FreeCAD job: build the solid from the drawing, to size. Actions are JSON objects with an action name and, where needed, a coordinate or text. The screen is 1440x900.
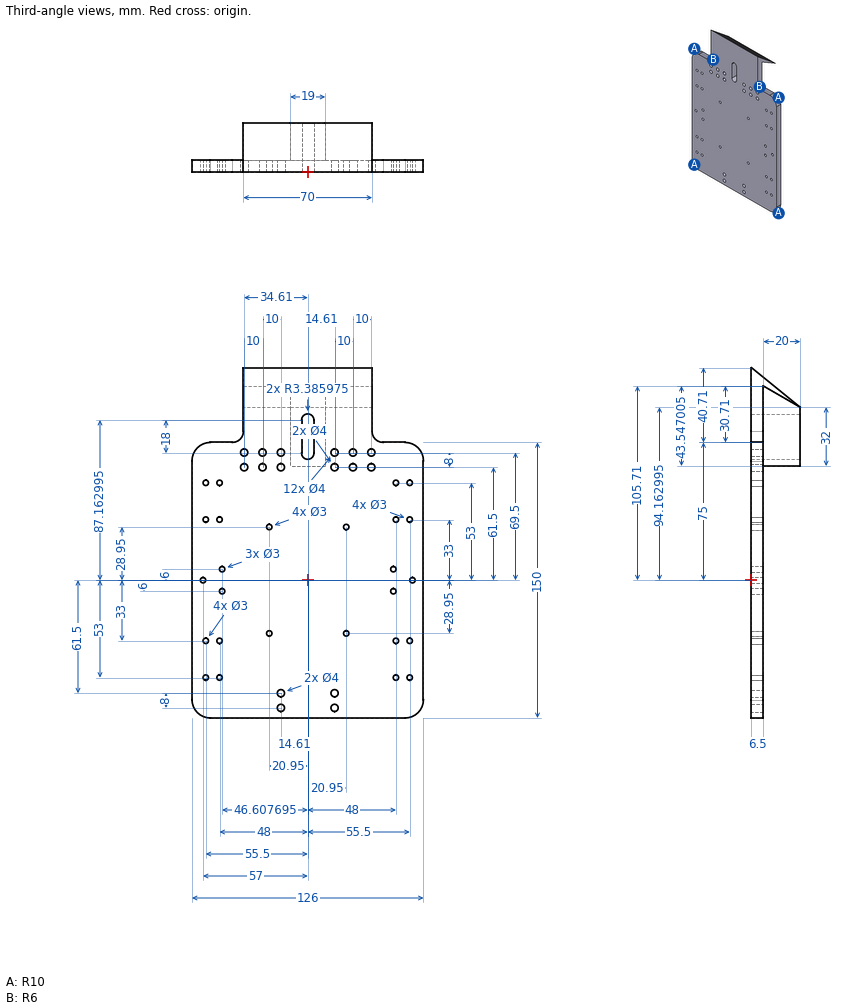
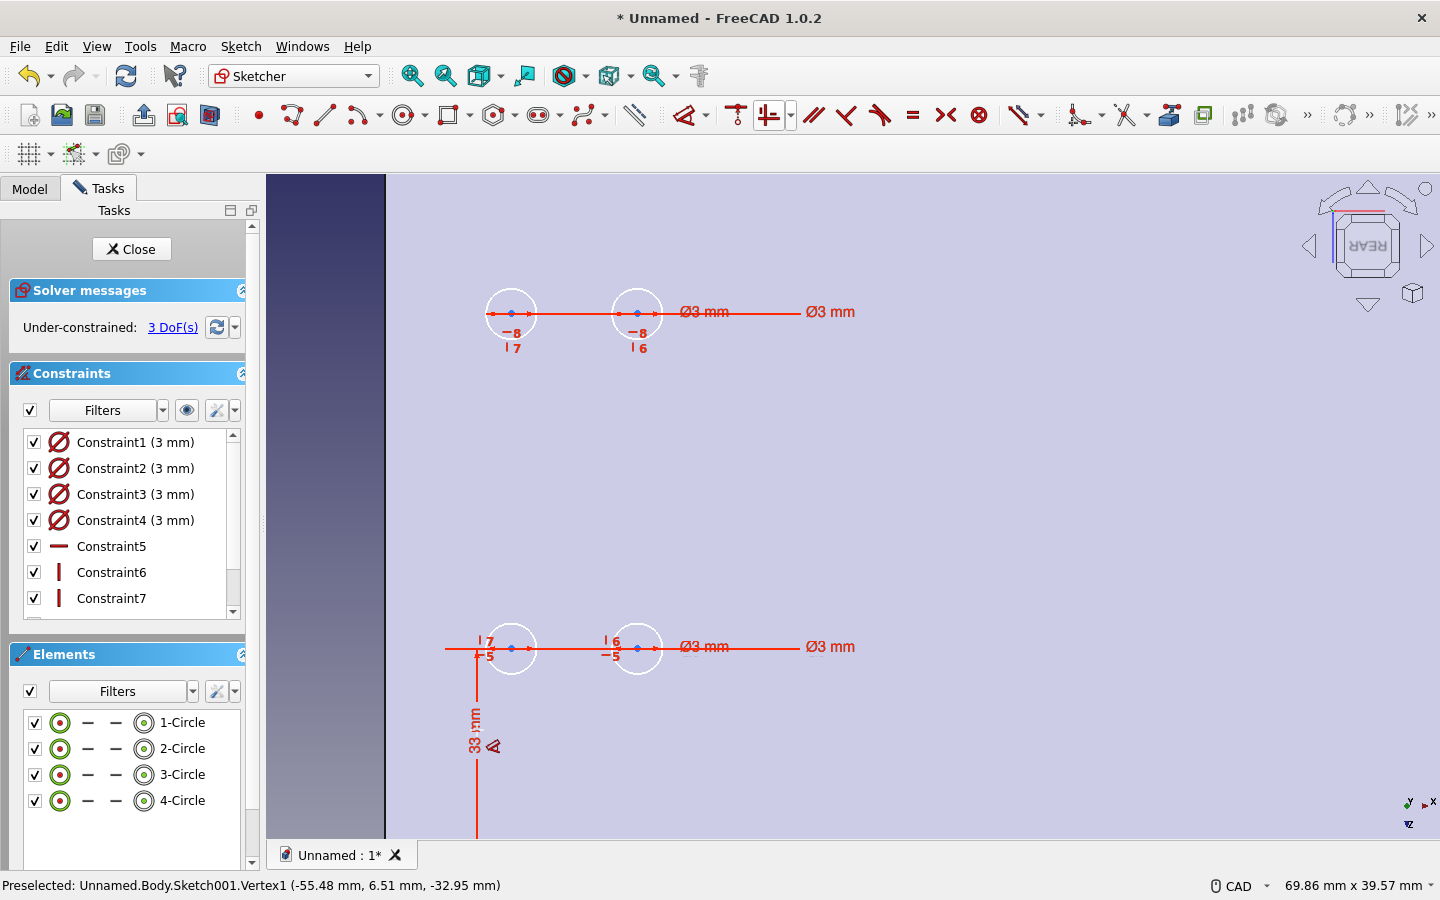
{"action": "left_click", "coordinate": [637, 649]}
{"action": "left_click", "coordinate": [956, 615]}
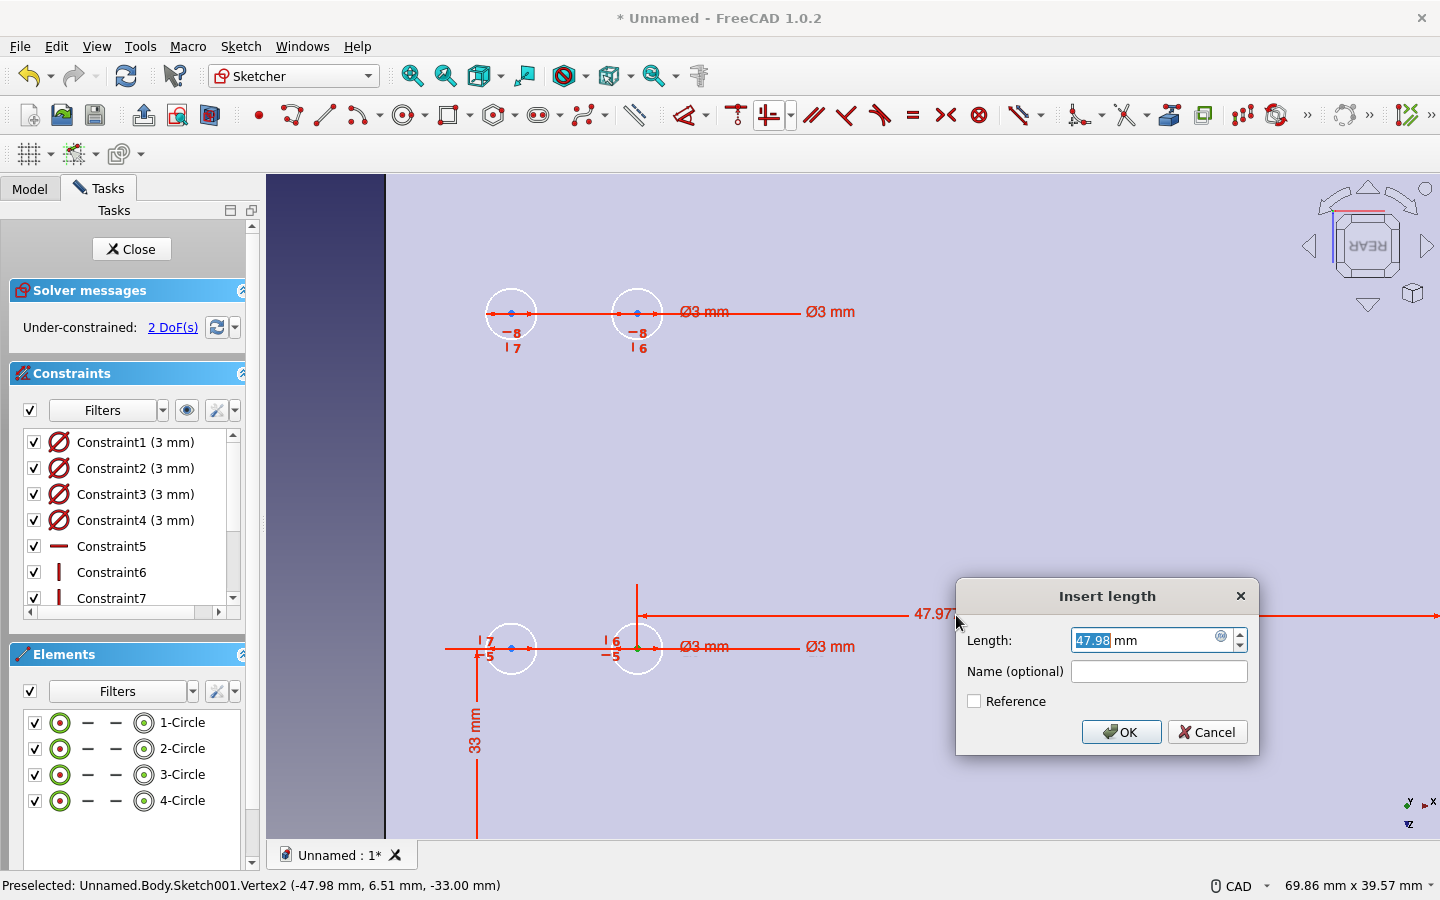
{"action": "type", "text": "48"}
{"action": "key", "text": "Return"}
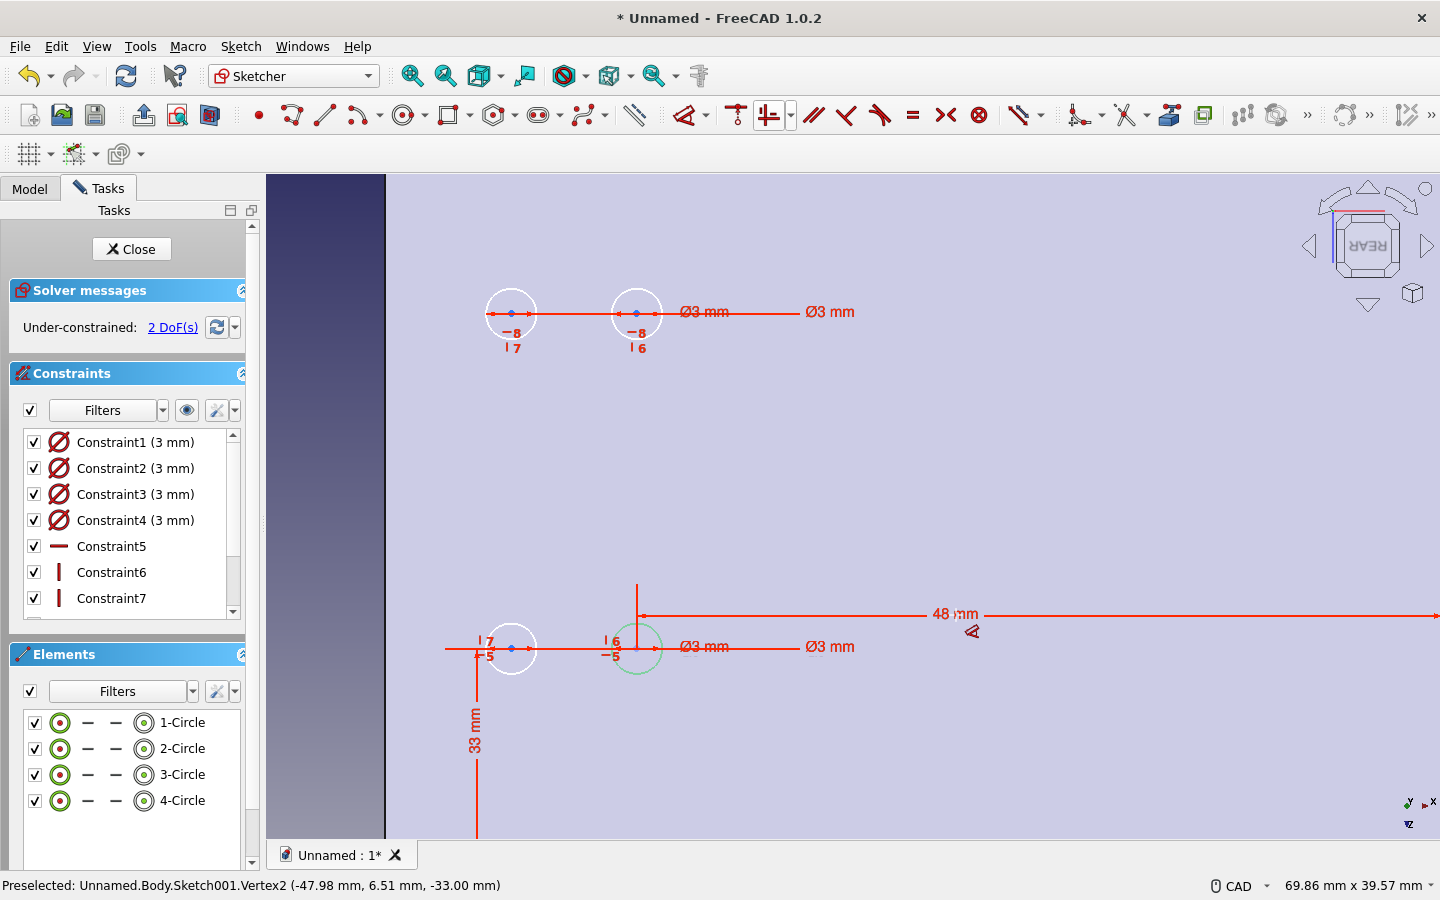
{"action": "left_click", "coordinate": [637, 314]}
{"action": "left_click", "coordinate": [603, 562]}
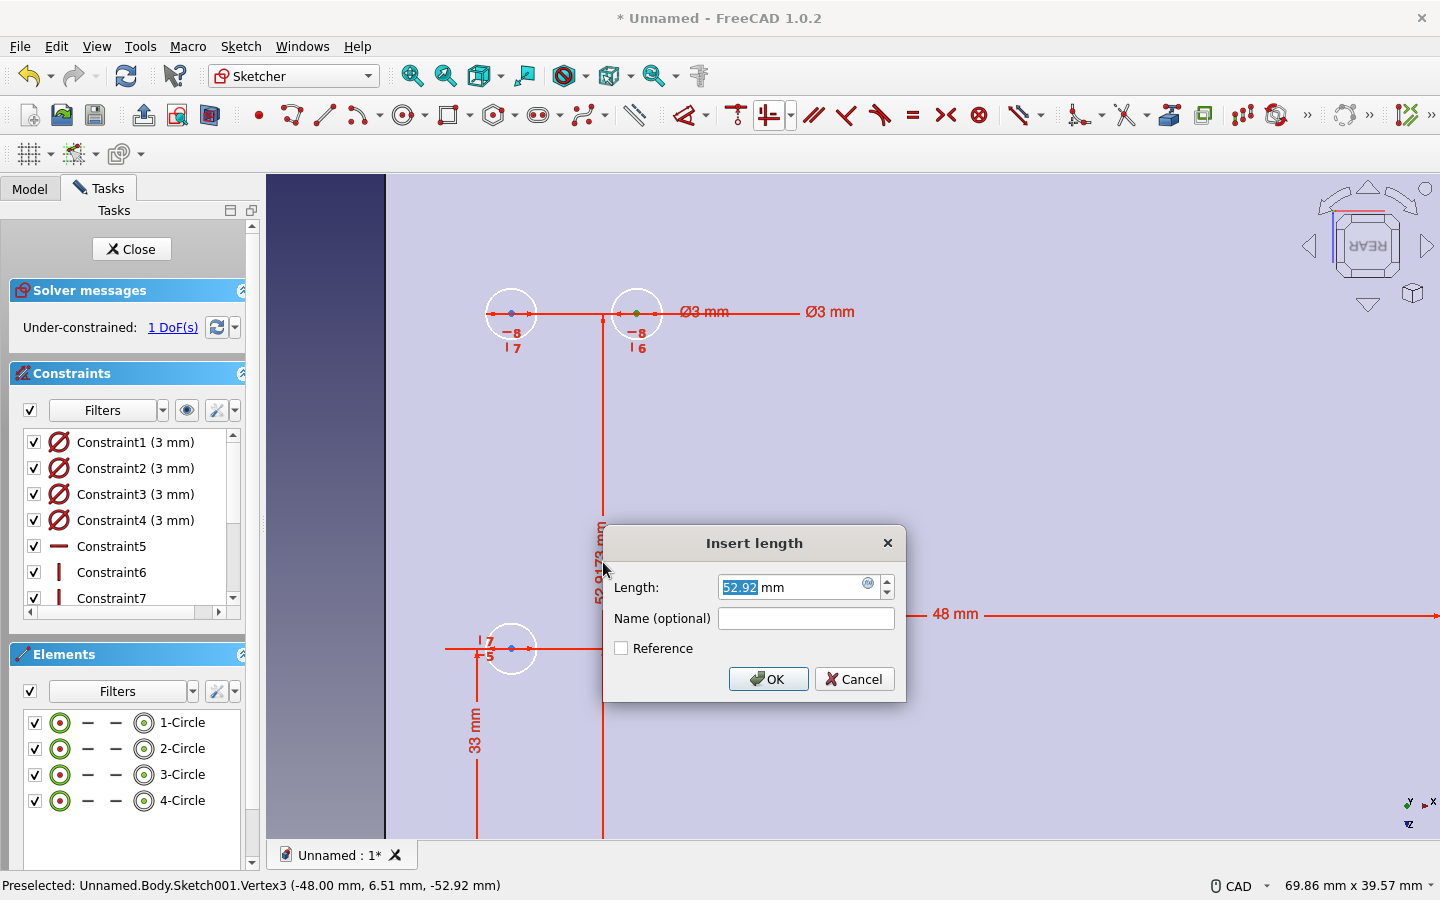
{"action": "type", "text": "53"}
{"action": "key", "text": "Return"}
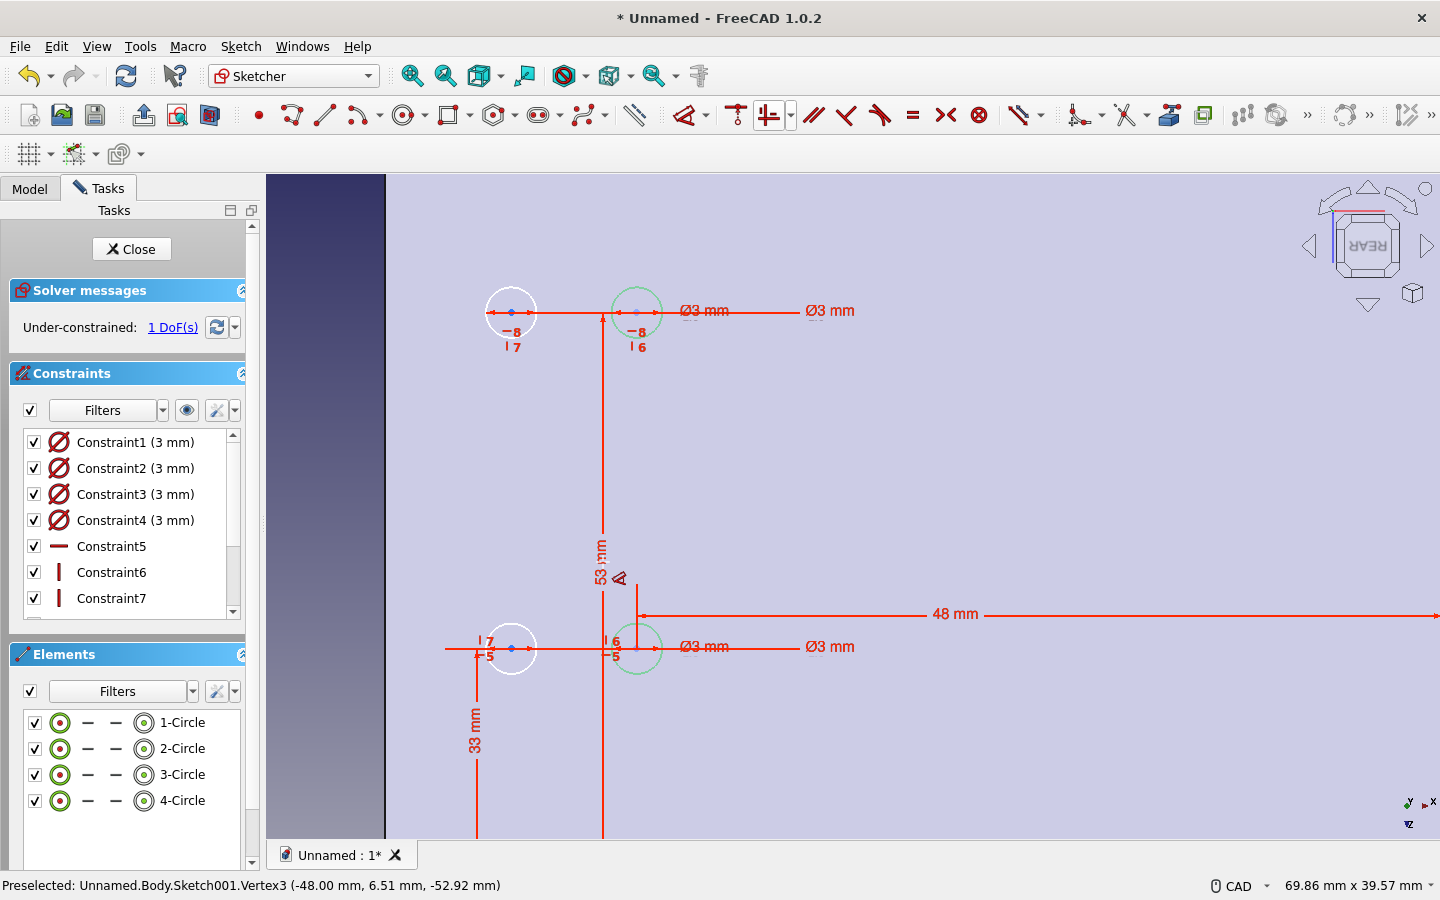
{"action": "left_click", "coordinate": [511, 649]}
{"action": "left_click", "coordinate": [718, 615]}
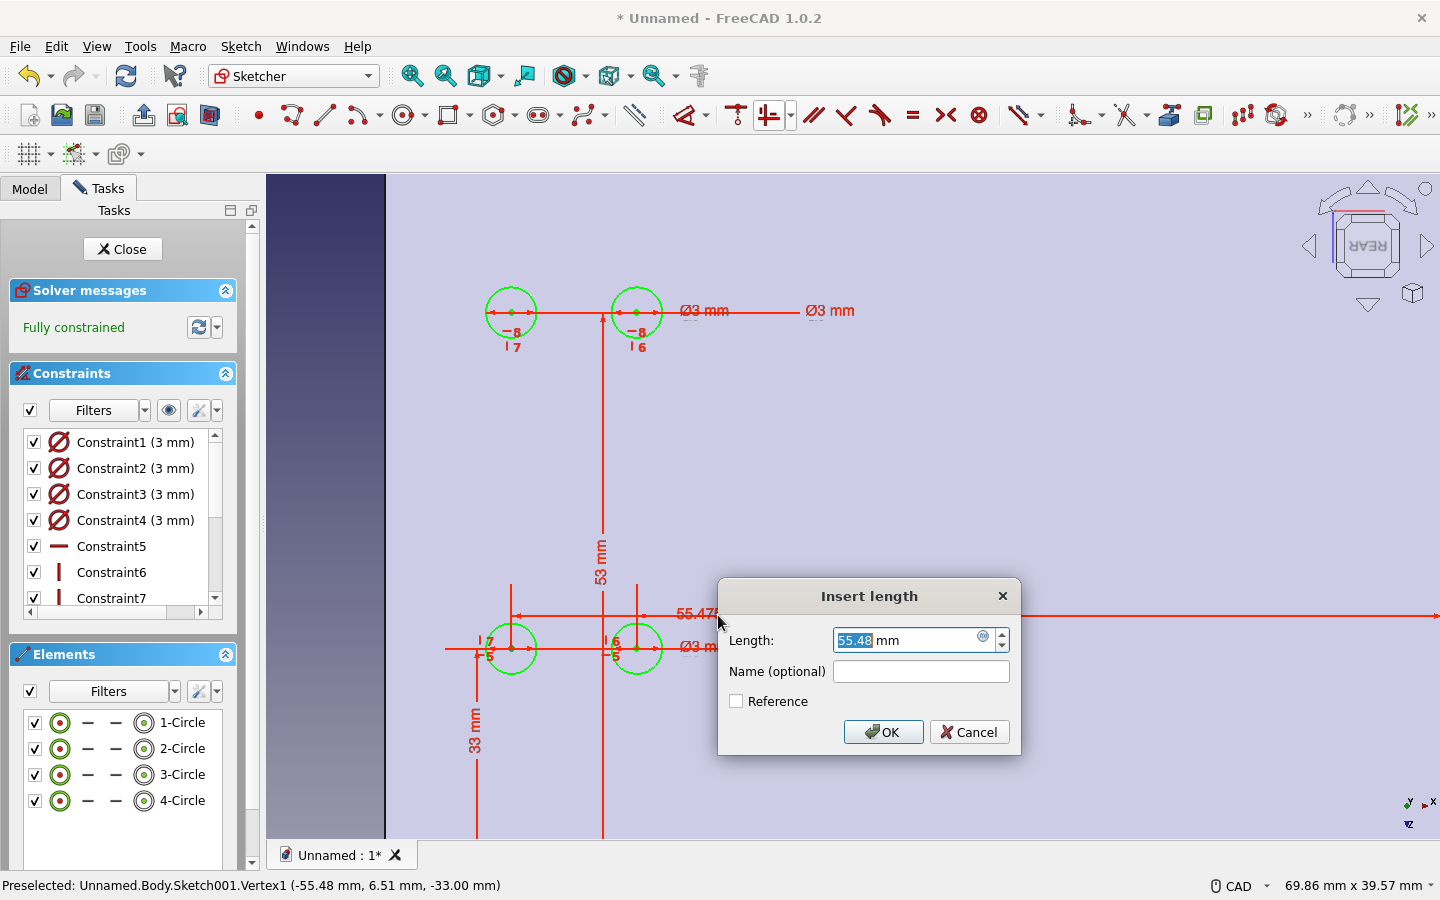
{"action": "type", "text": "55.5"}
{"action": "key", "text": "Return"}
{"action": "key", "text": "Escape"}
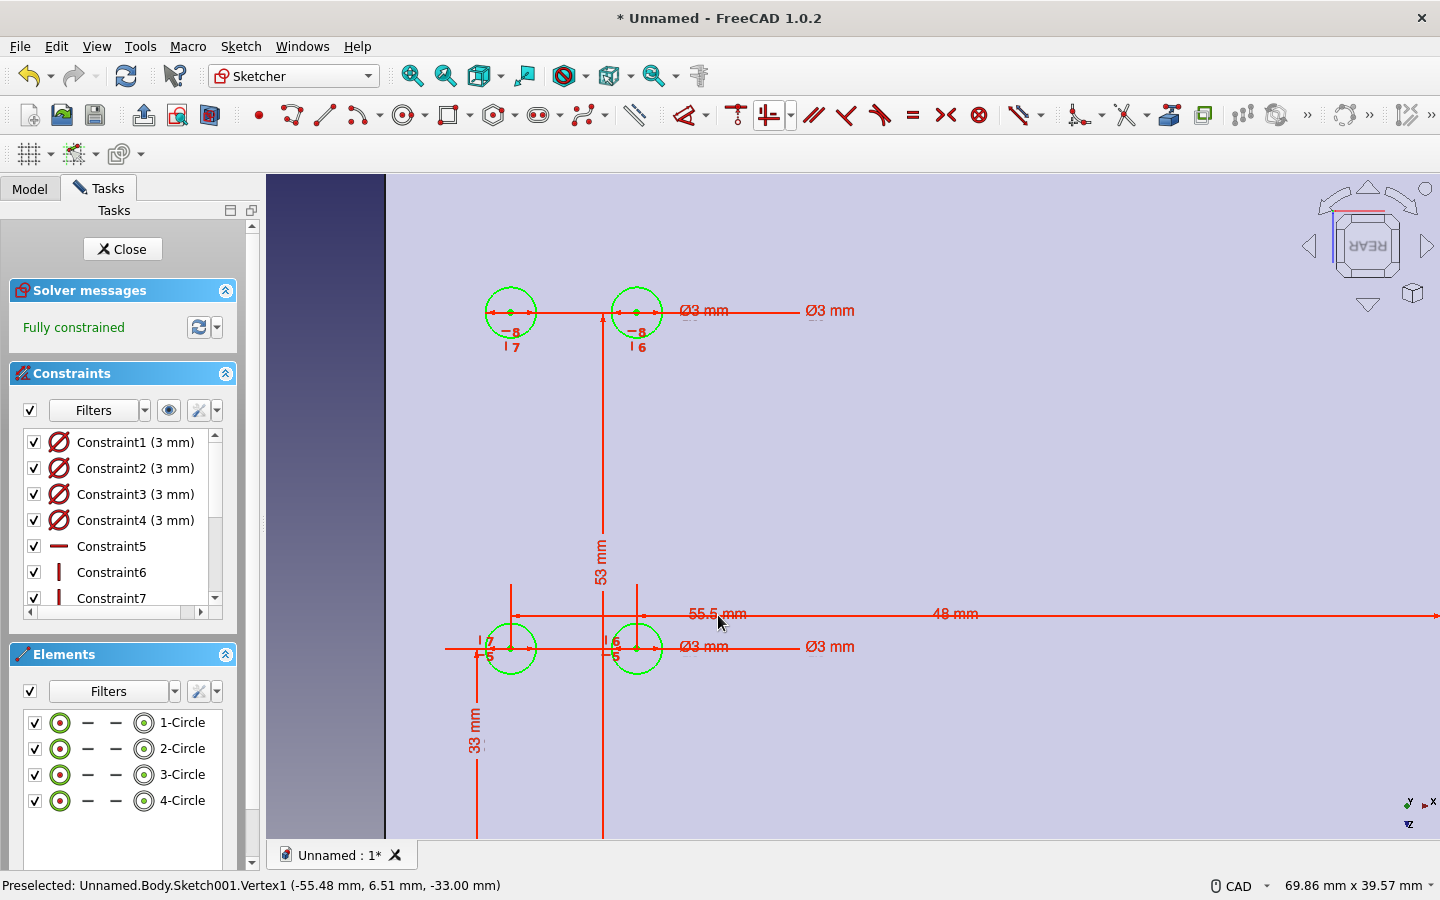
{"action": "left_click", "coordinate": [123, 249]}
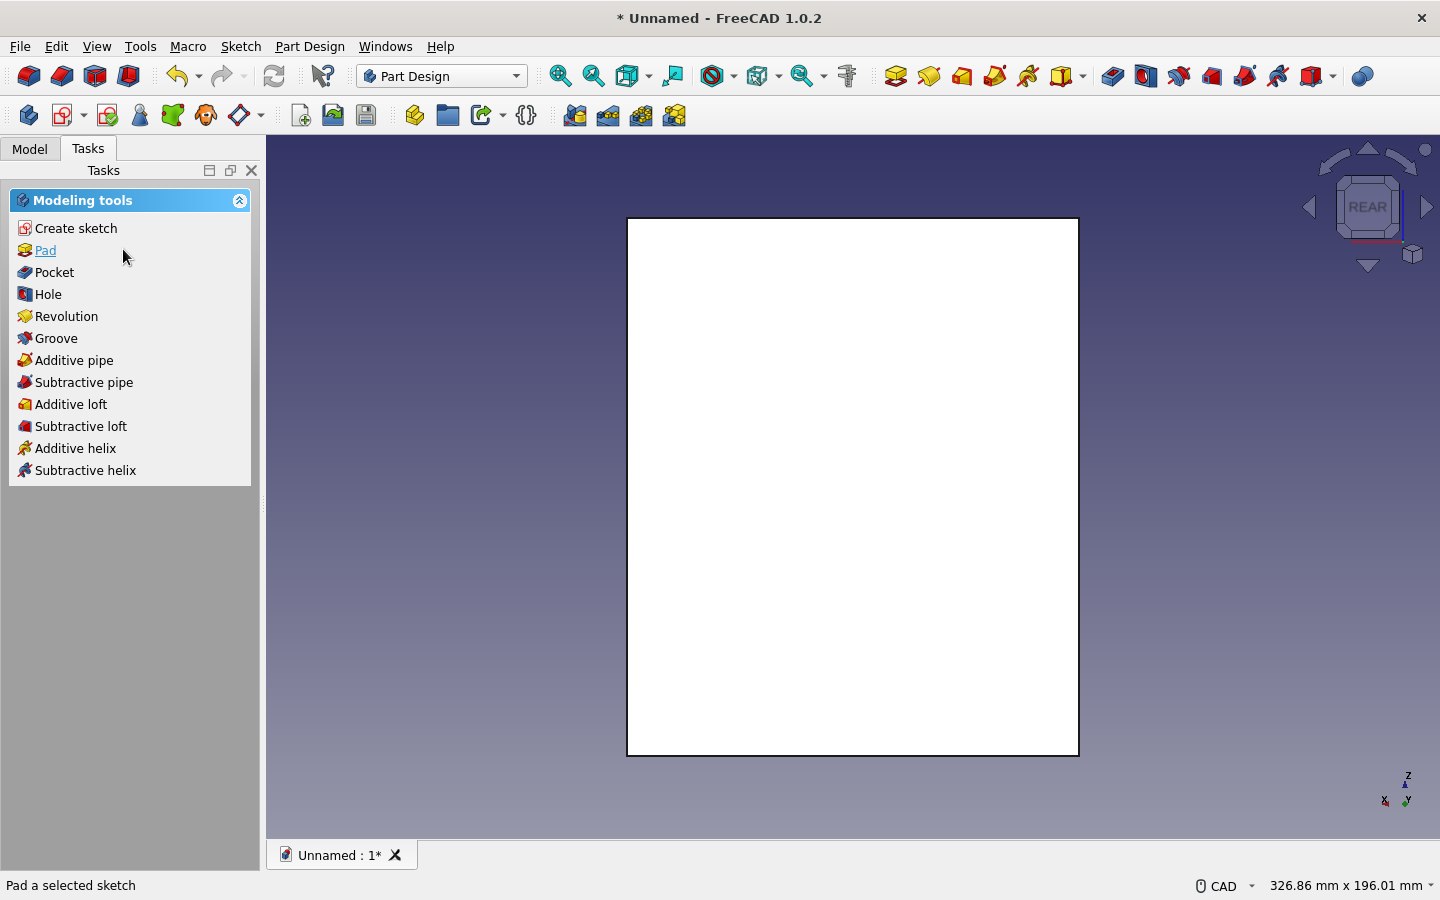
{"action": "left_click", "coordinate": [1113, 76]}